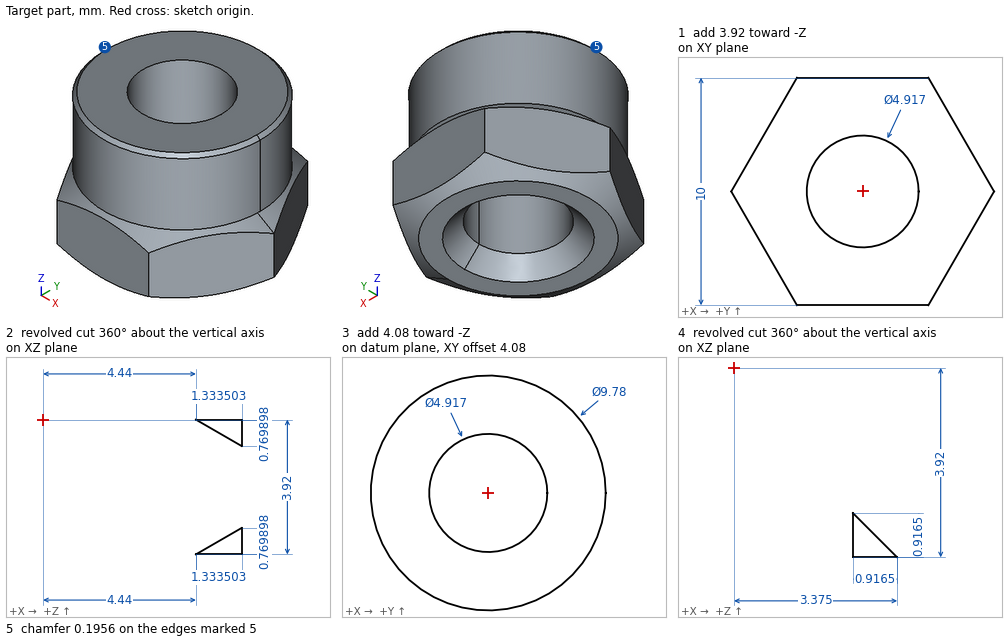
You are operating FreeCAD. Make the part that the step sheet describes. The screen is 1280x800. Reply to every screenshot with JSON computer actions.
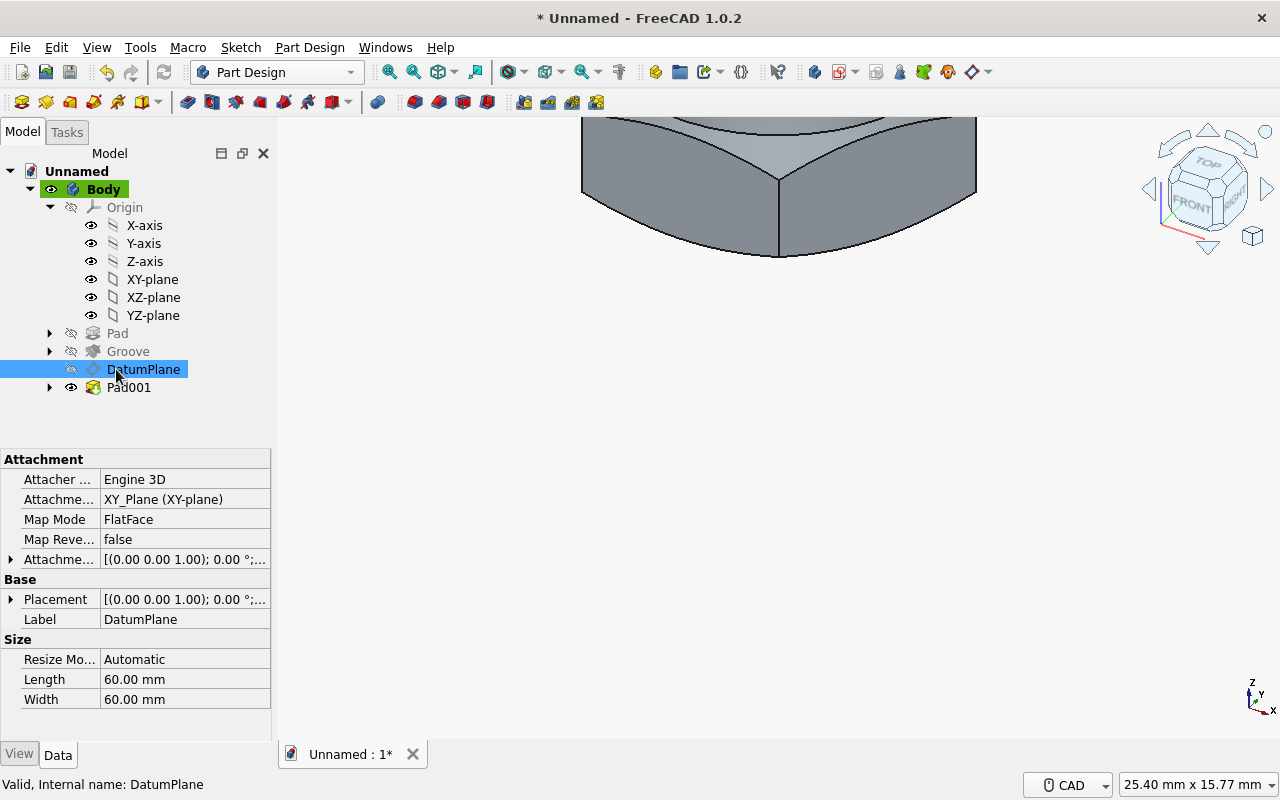
{"action": "key", "text": "v f"}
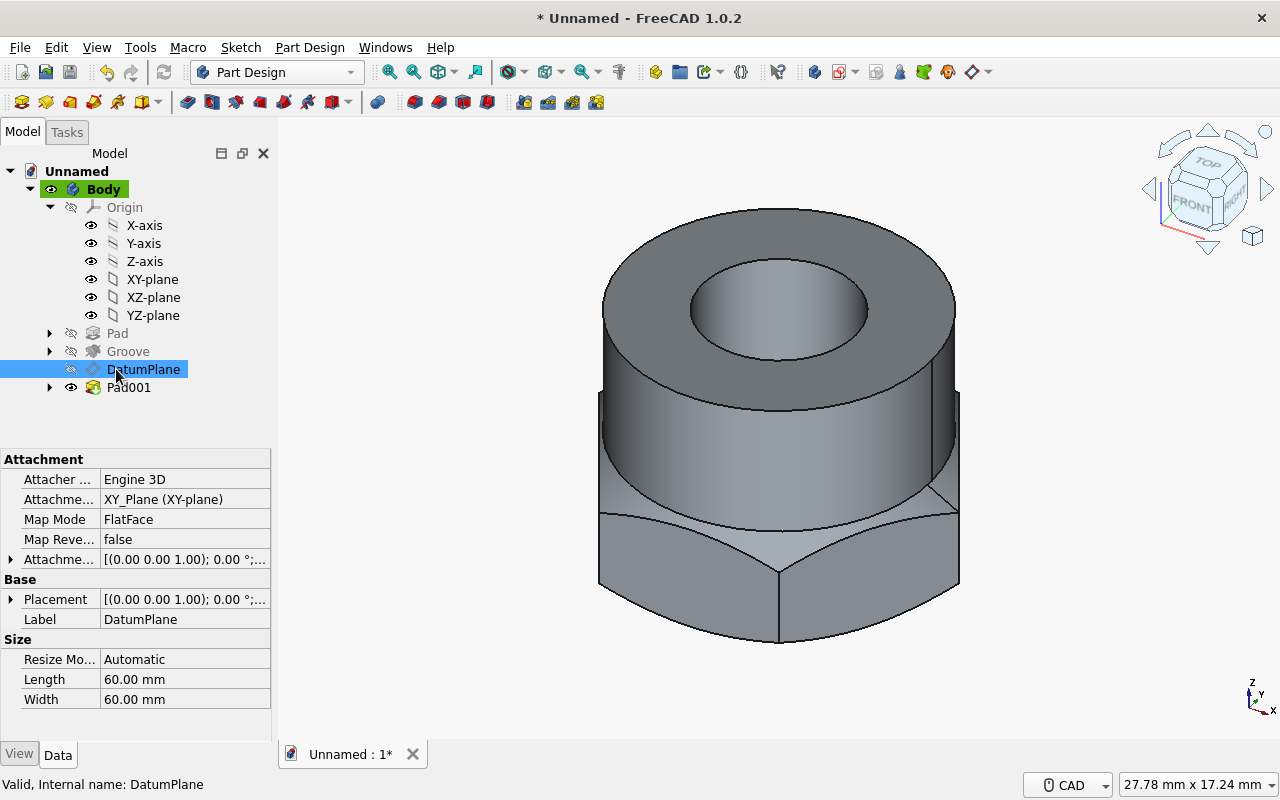
{"action": "left_click", "coordinate": [318, 699]}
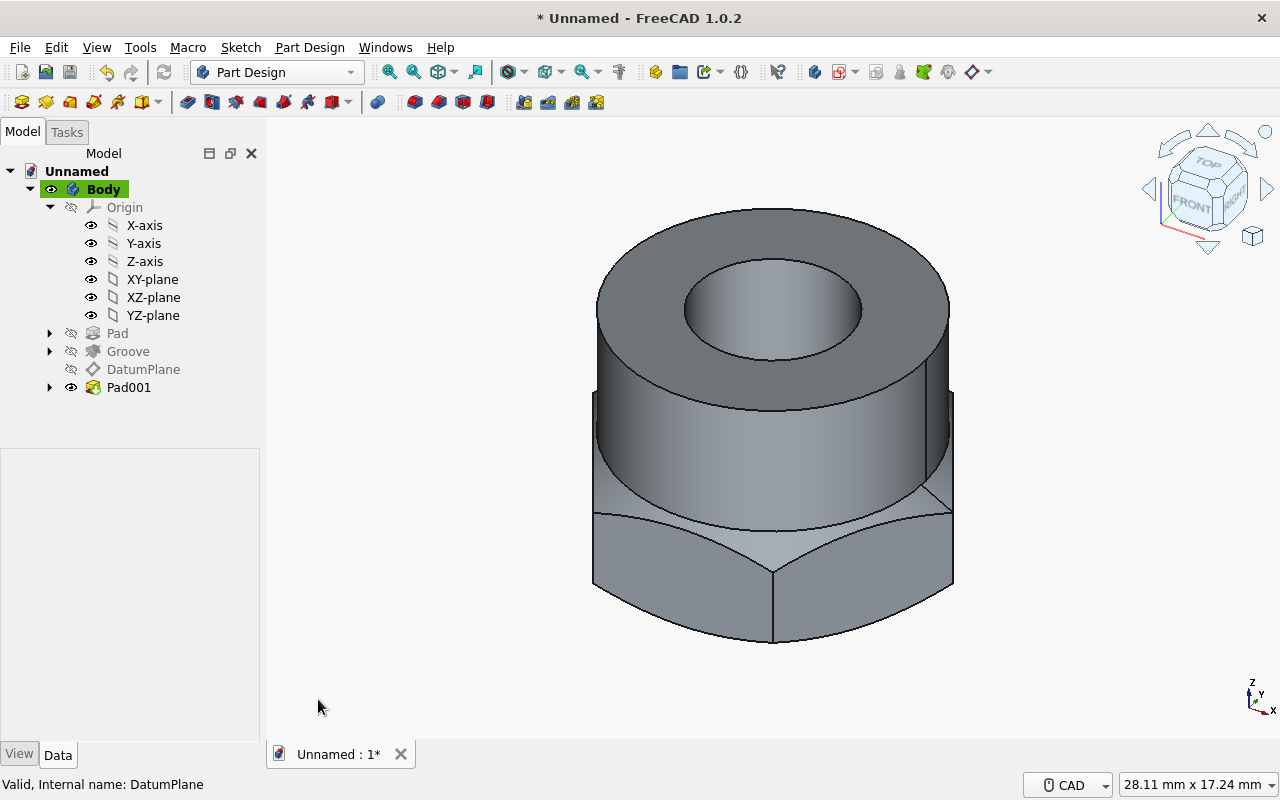
{"action": "left_click", "coordinate": [840, 72]}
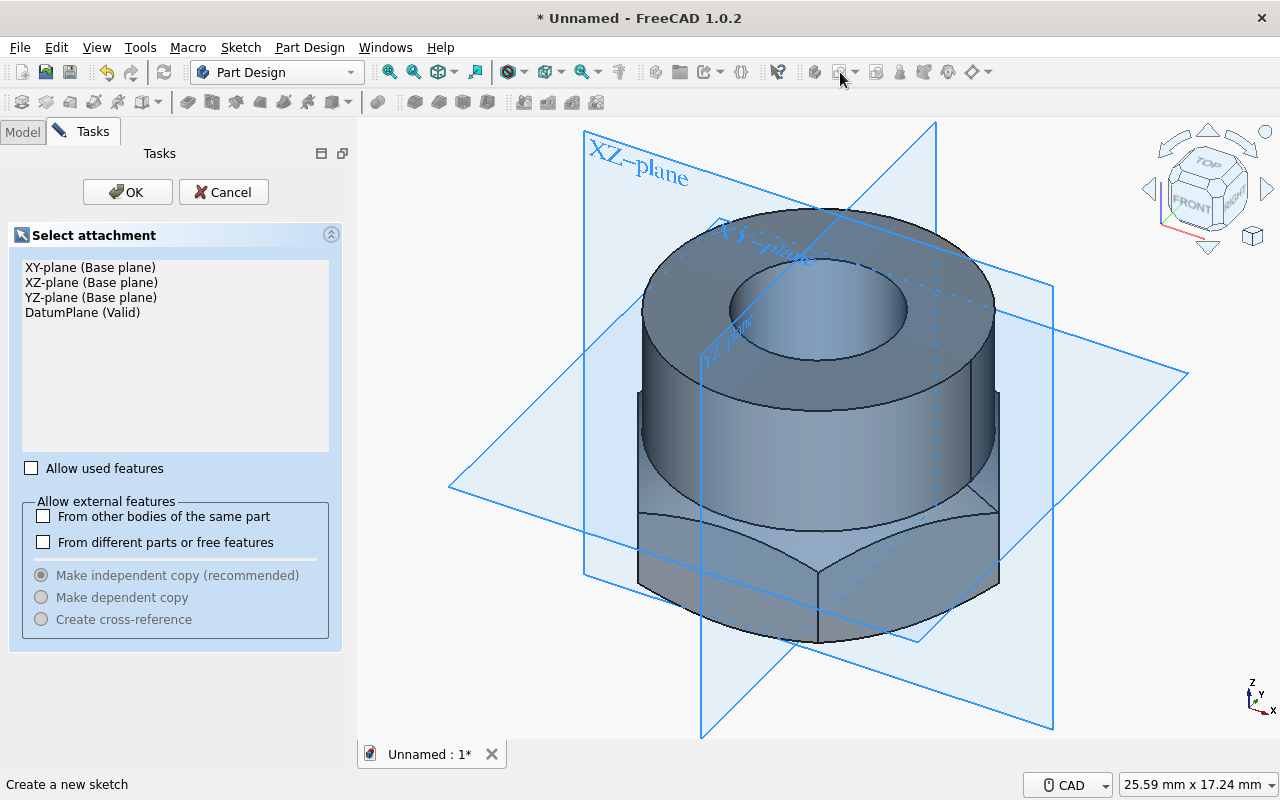
{"action": "left_click", "coordinate": [82, 282]}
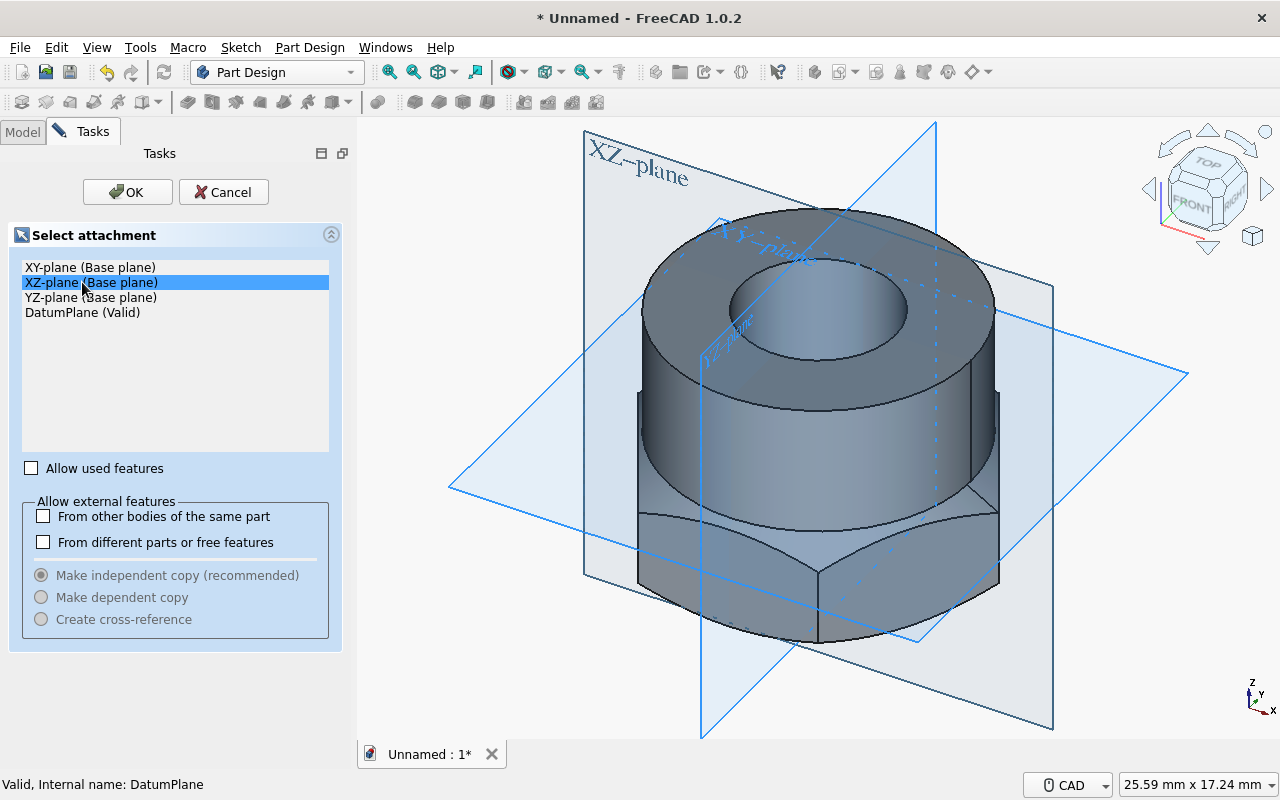
{"action": "left_click", "coordinate": [128, 192]}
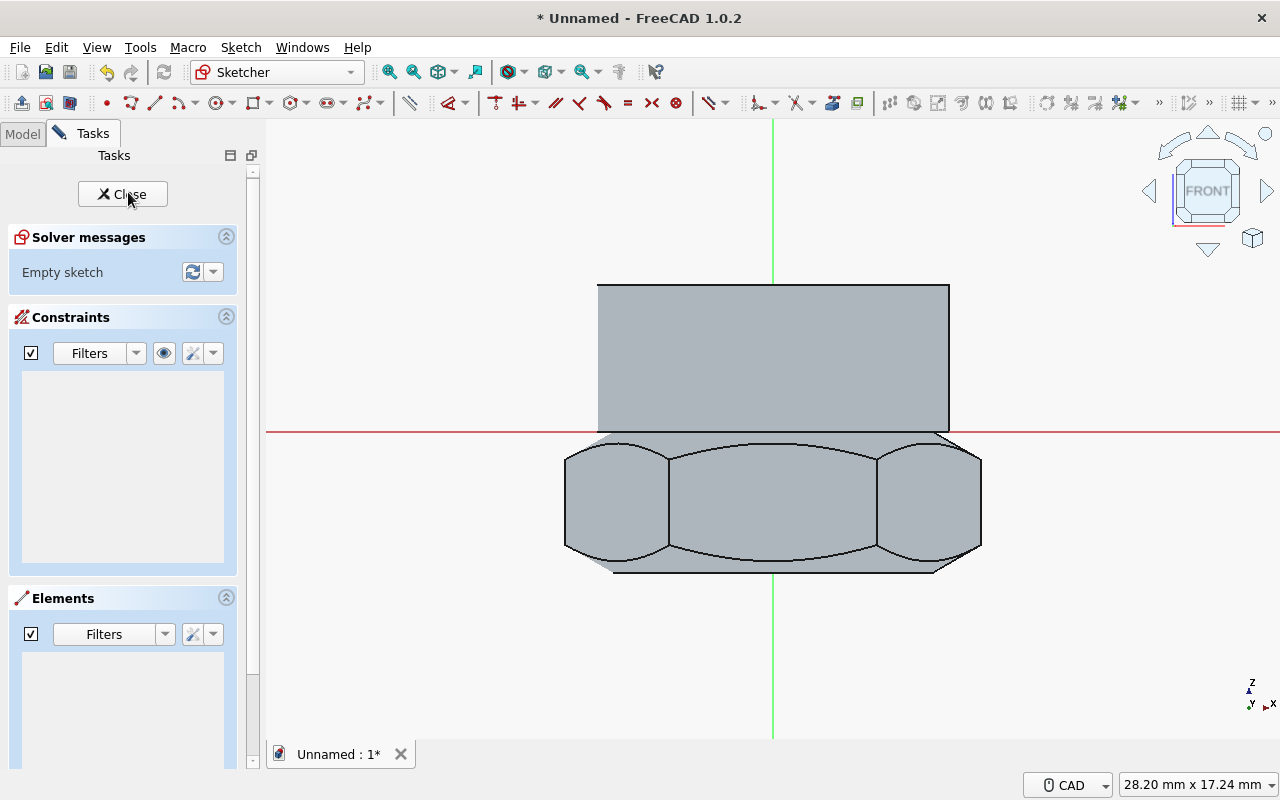
{"action": "key", "text": "q s"}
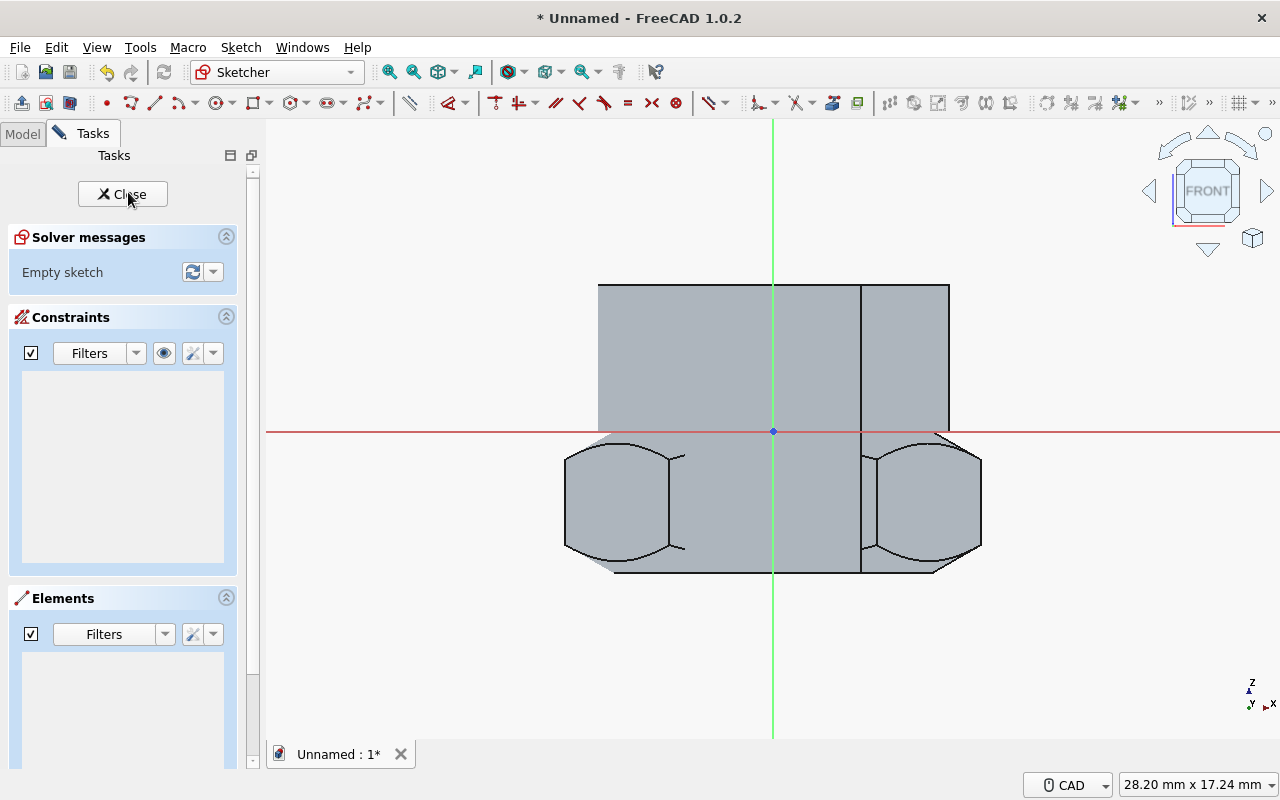
{"action": "scroll", "coordinate": [895, 569], "scroll_direction": "up", "scroll_amount": 12}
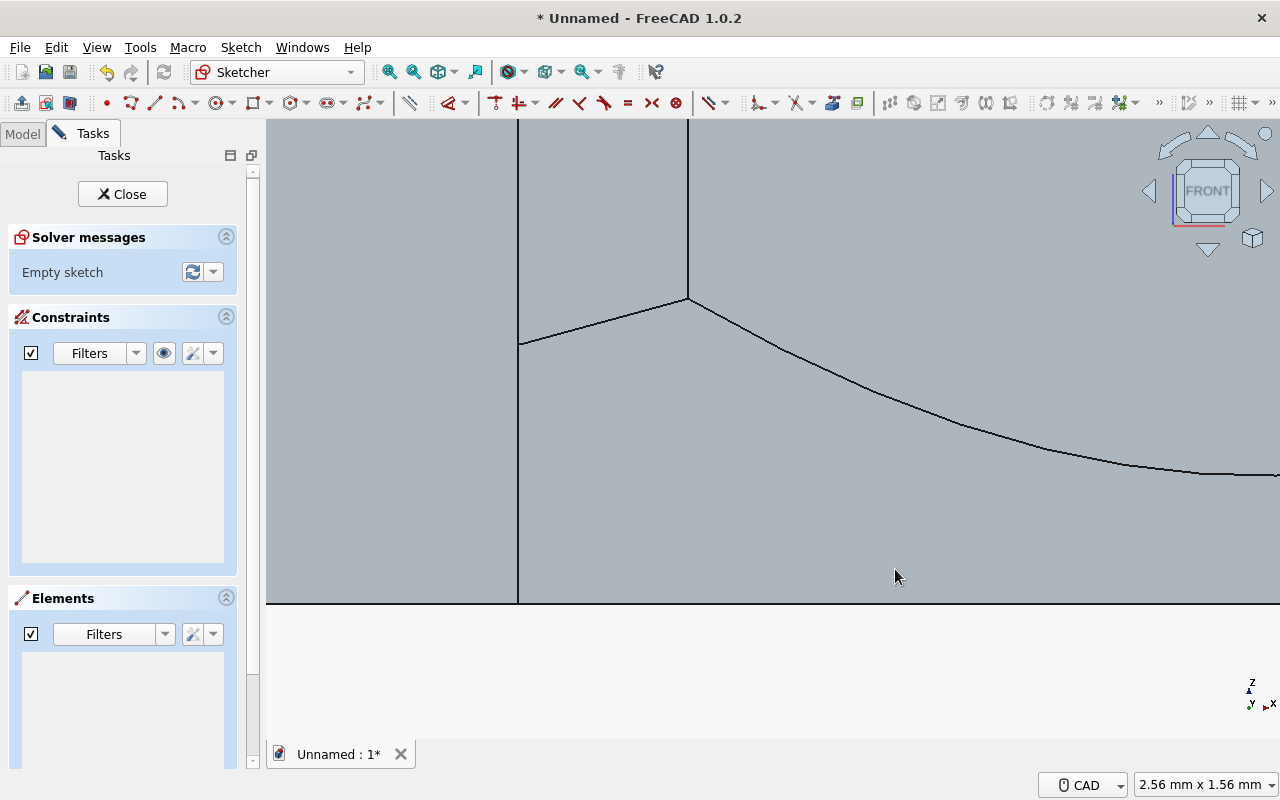
{"action": "key", "text": "g m"}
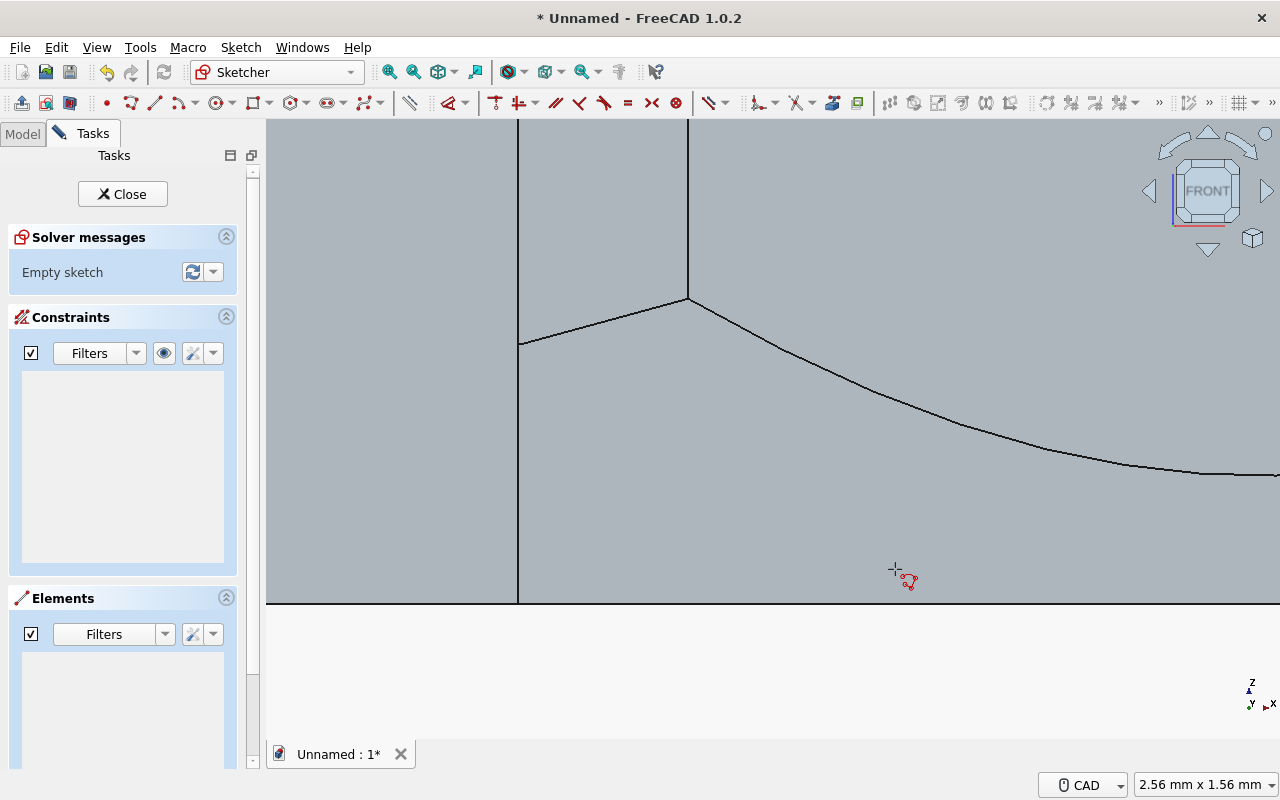
{"action": "left_click", "coordinate": [518, 241]}
{"action": "left_click", "coordinate": [882, 604]}
{"action": "left_click", "coordinate": [518, 604]}
{"action": "left_click", "coordinate": [518, 242]}
{"action": "key", "text": "Escape"}
{"action": "key", "text": "Escape"}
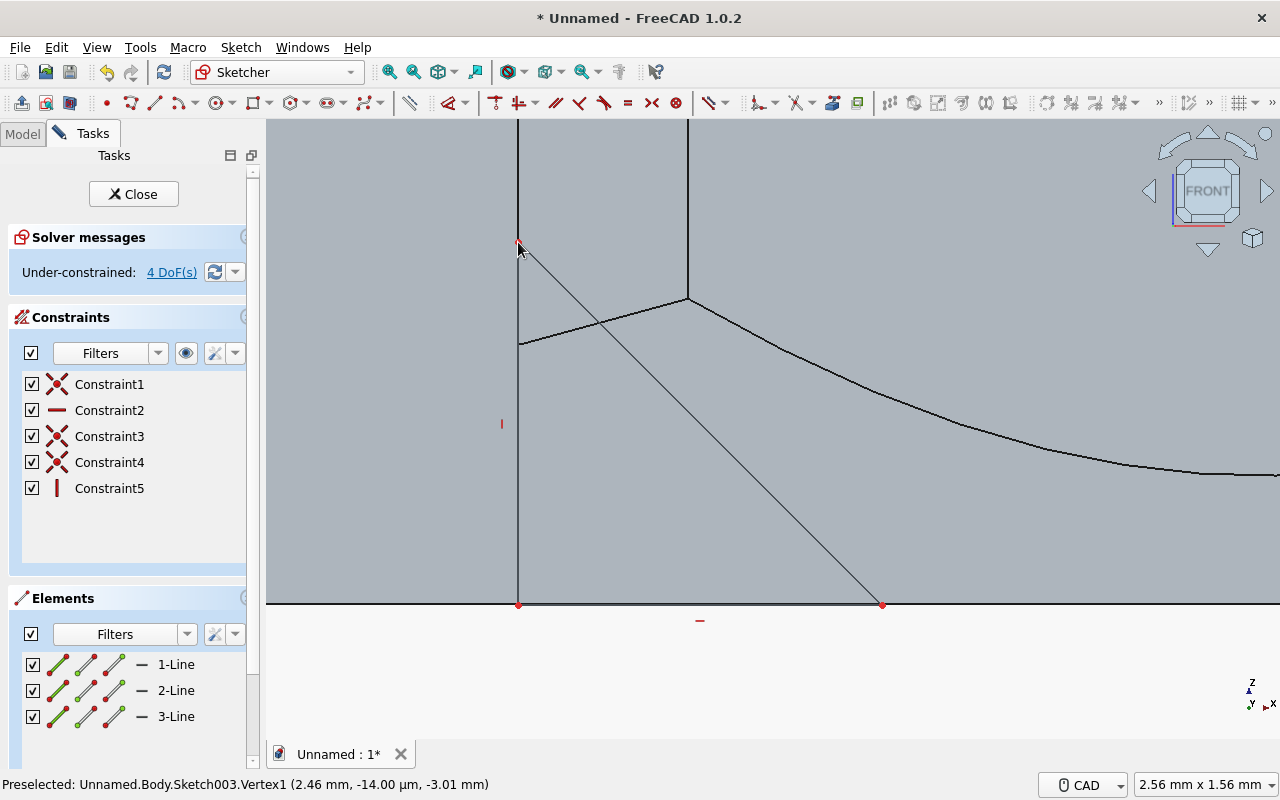
{"action": "left_click", "coordinate": [448, 104]}